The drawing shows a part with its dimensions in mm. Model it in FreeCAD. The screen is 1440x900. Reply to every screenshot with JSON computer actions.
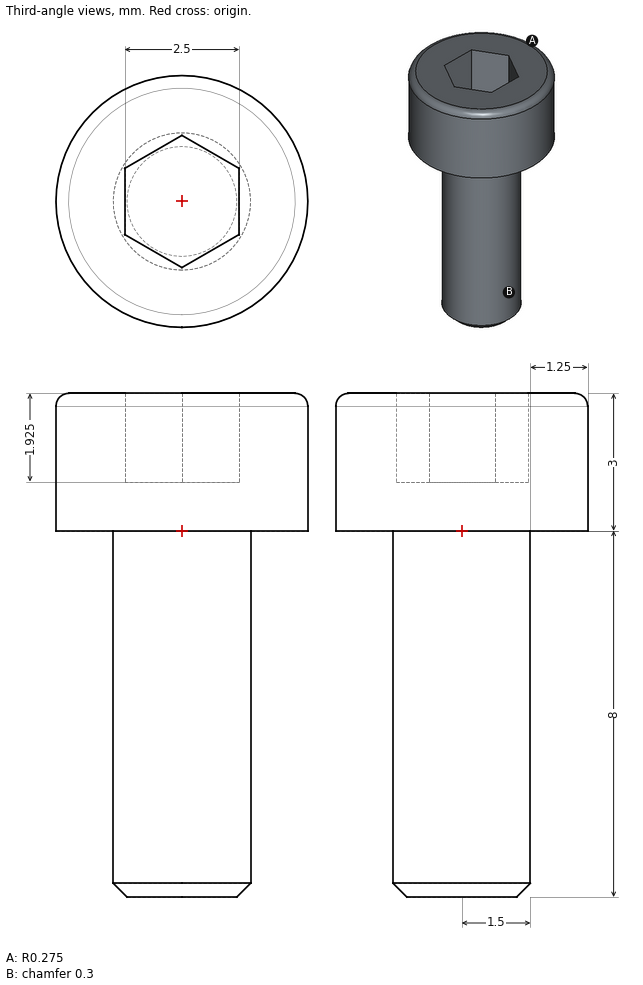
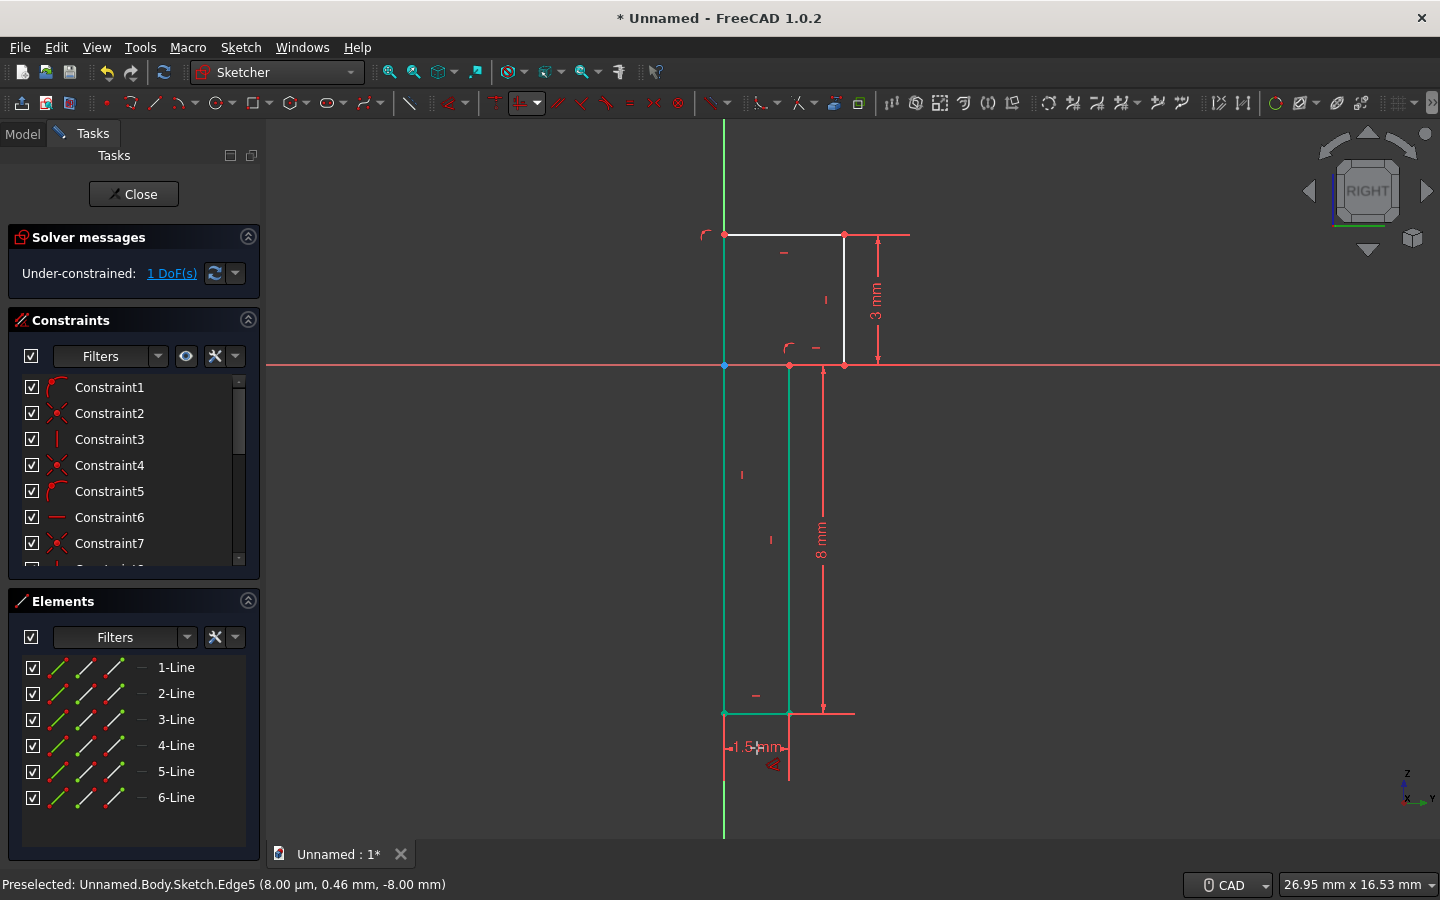
{"action": "left_click", "coordinate": [806, 365]}
{"action": "left_click", "coordinate": [817, 331]}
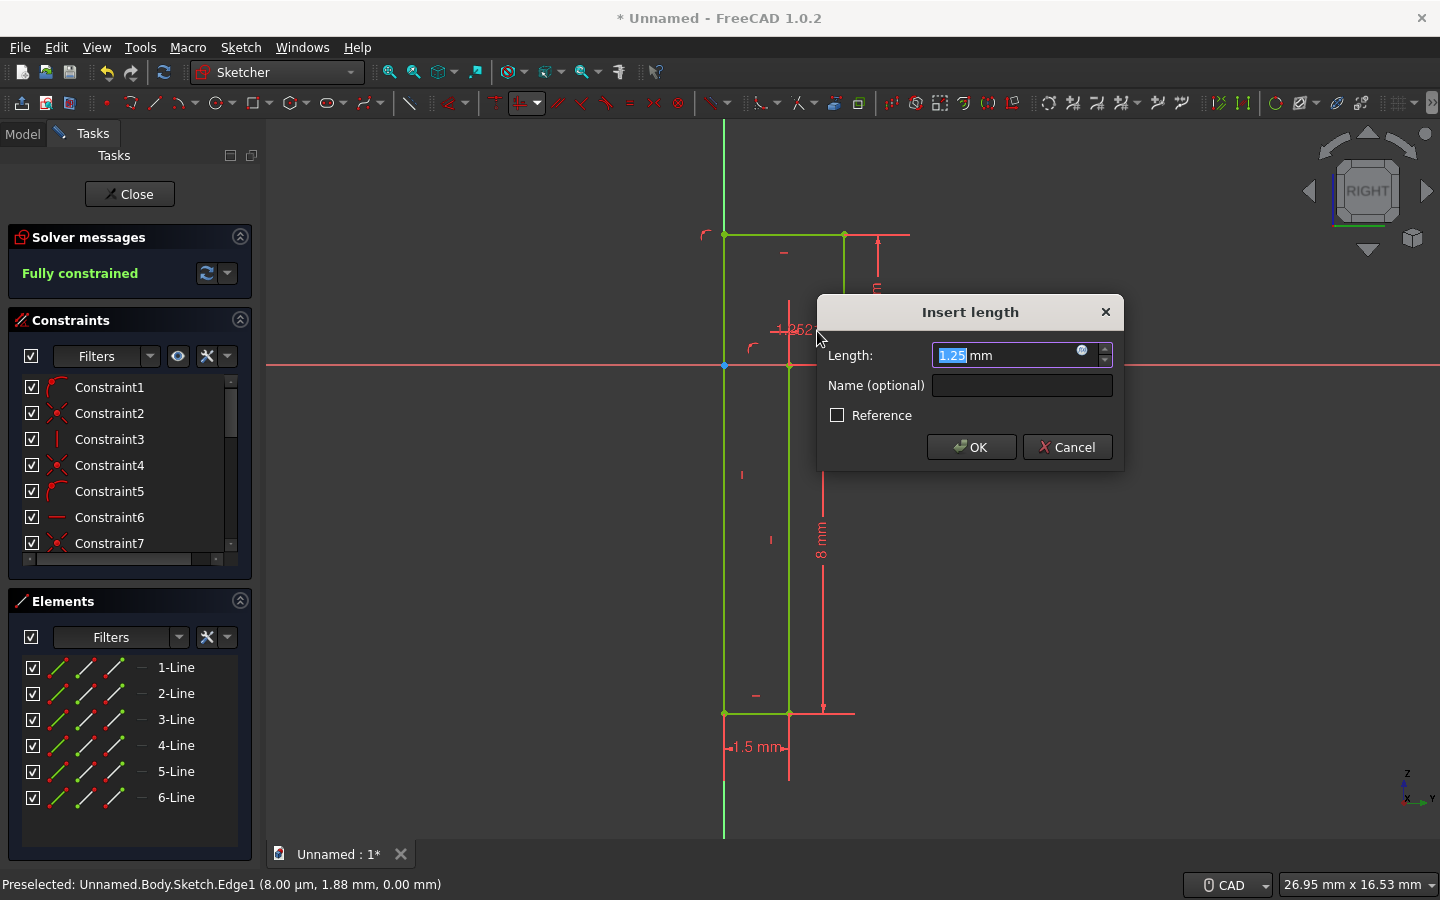
{"action": "type", "text": "1.25"}
{"action": "key", "text": "Return"}
{"action": "key", "text": "Escape"}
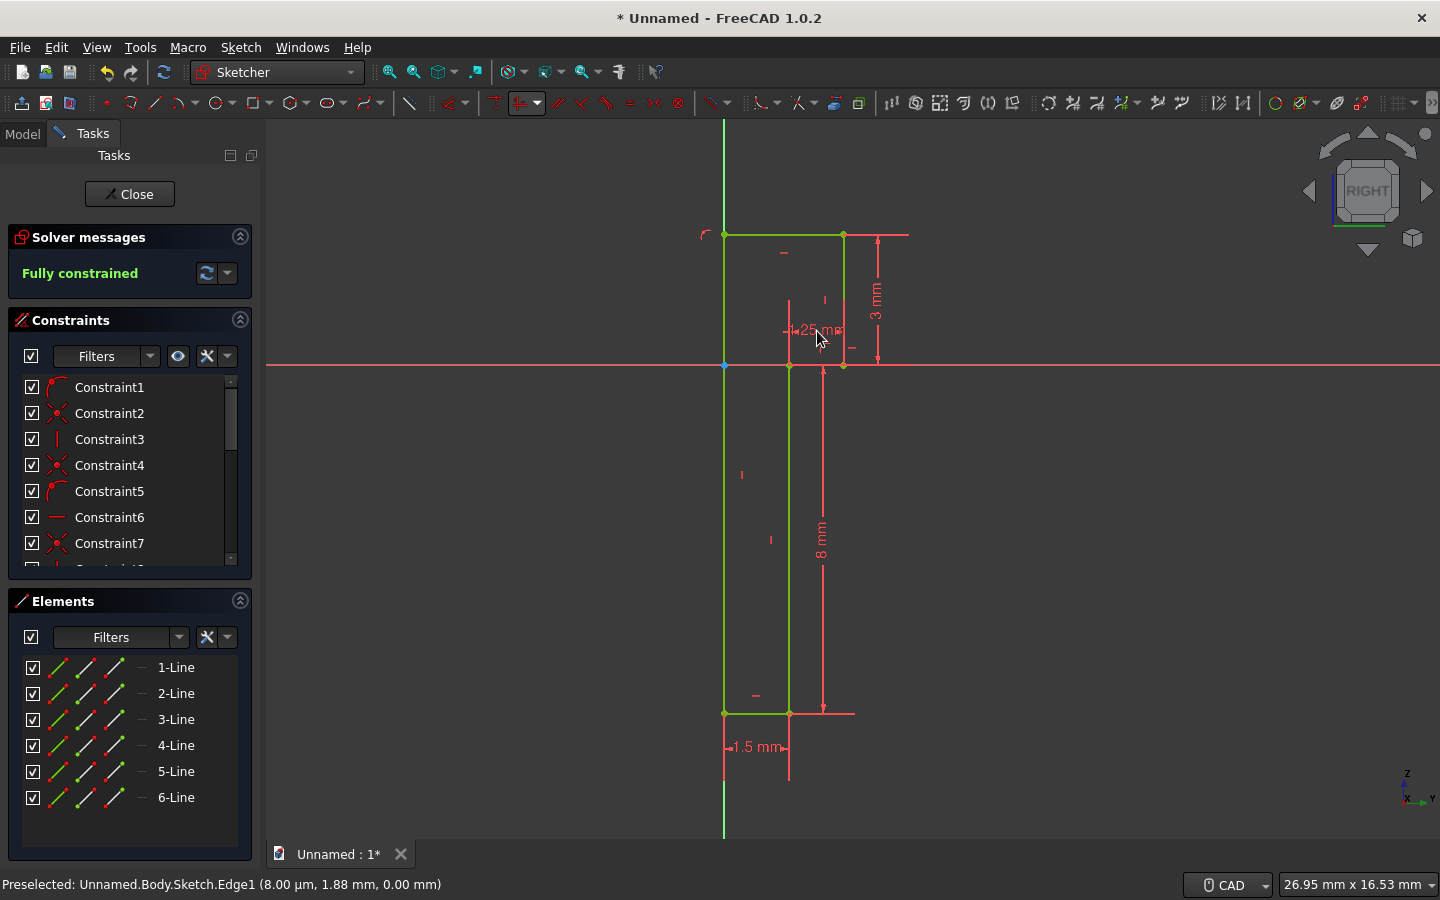
{"action": "left_click", "coordinate": [130, 194]}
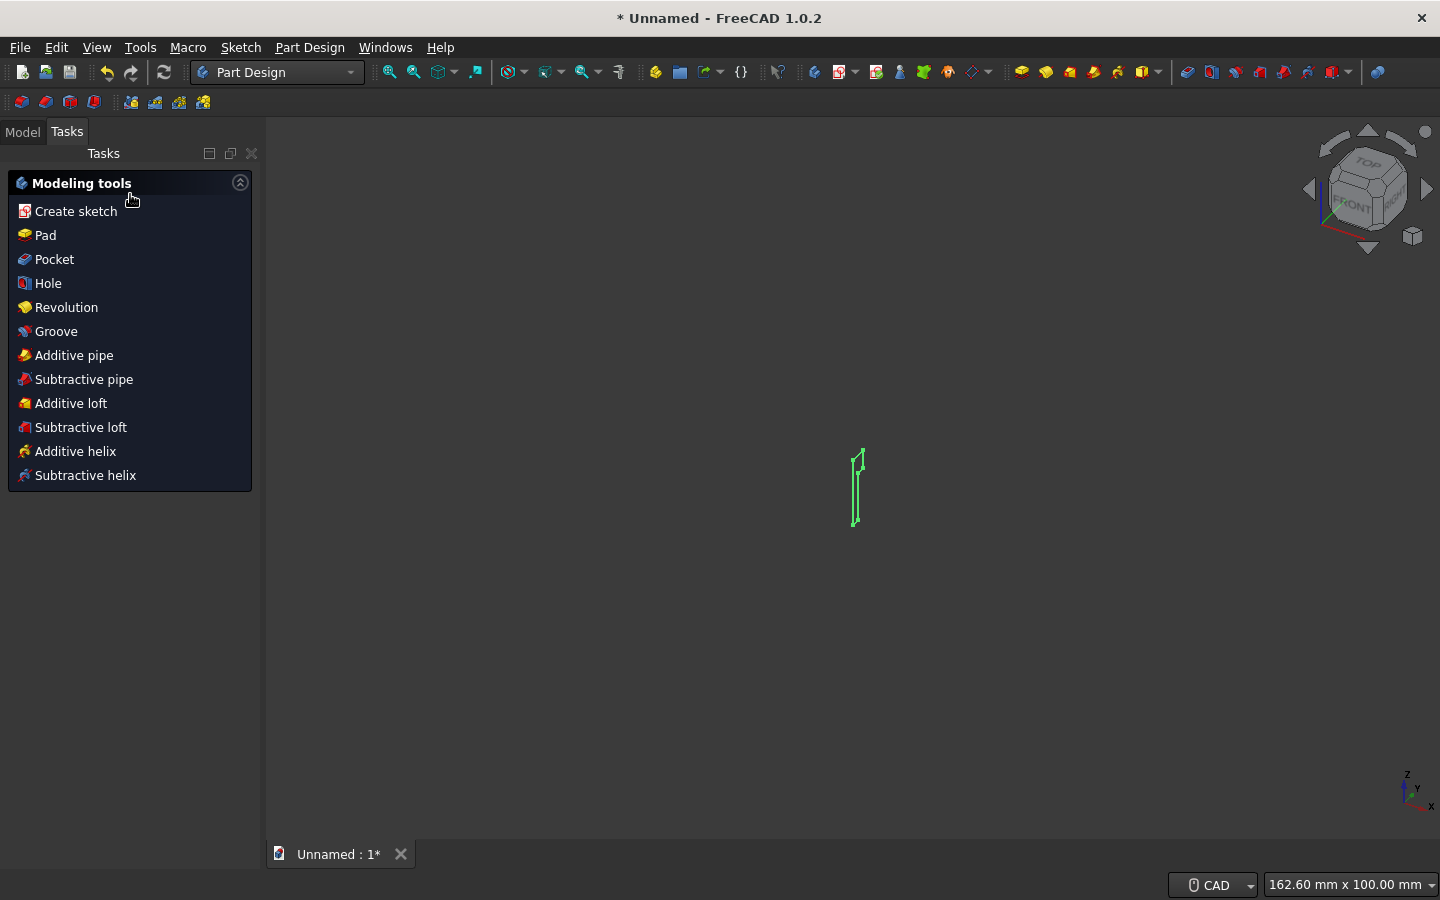
{"action": "left_click", "coordinate": [1046, 72]}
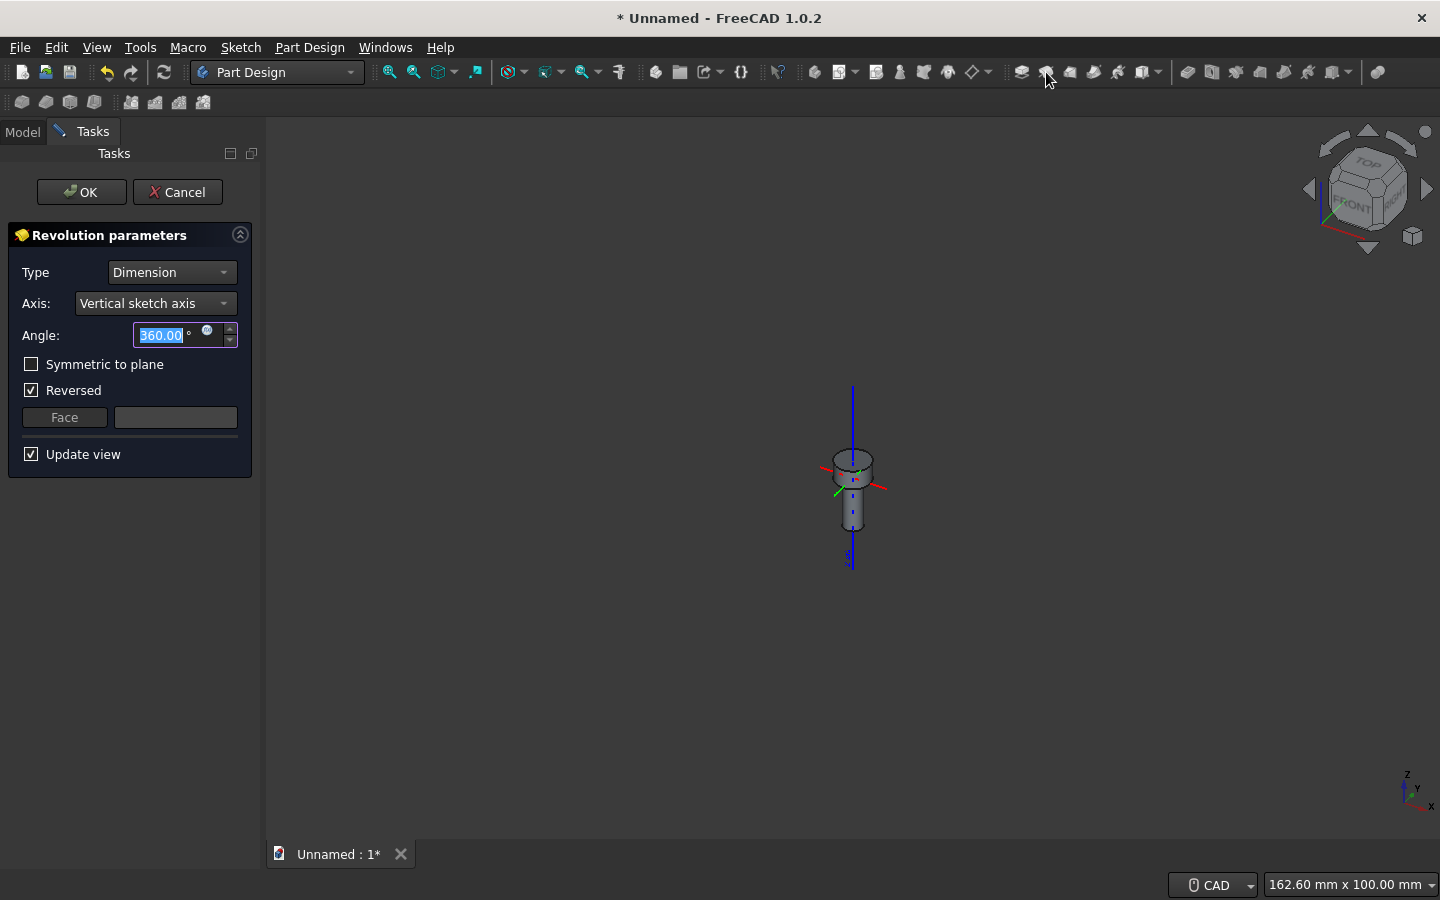
{"action": "left_click", "coordinate": [82, 192]}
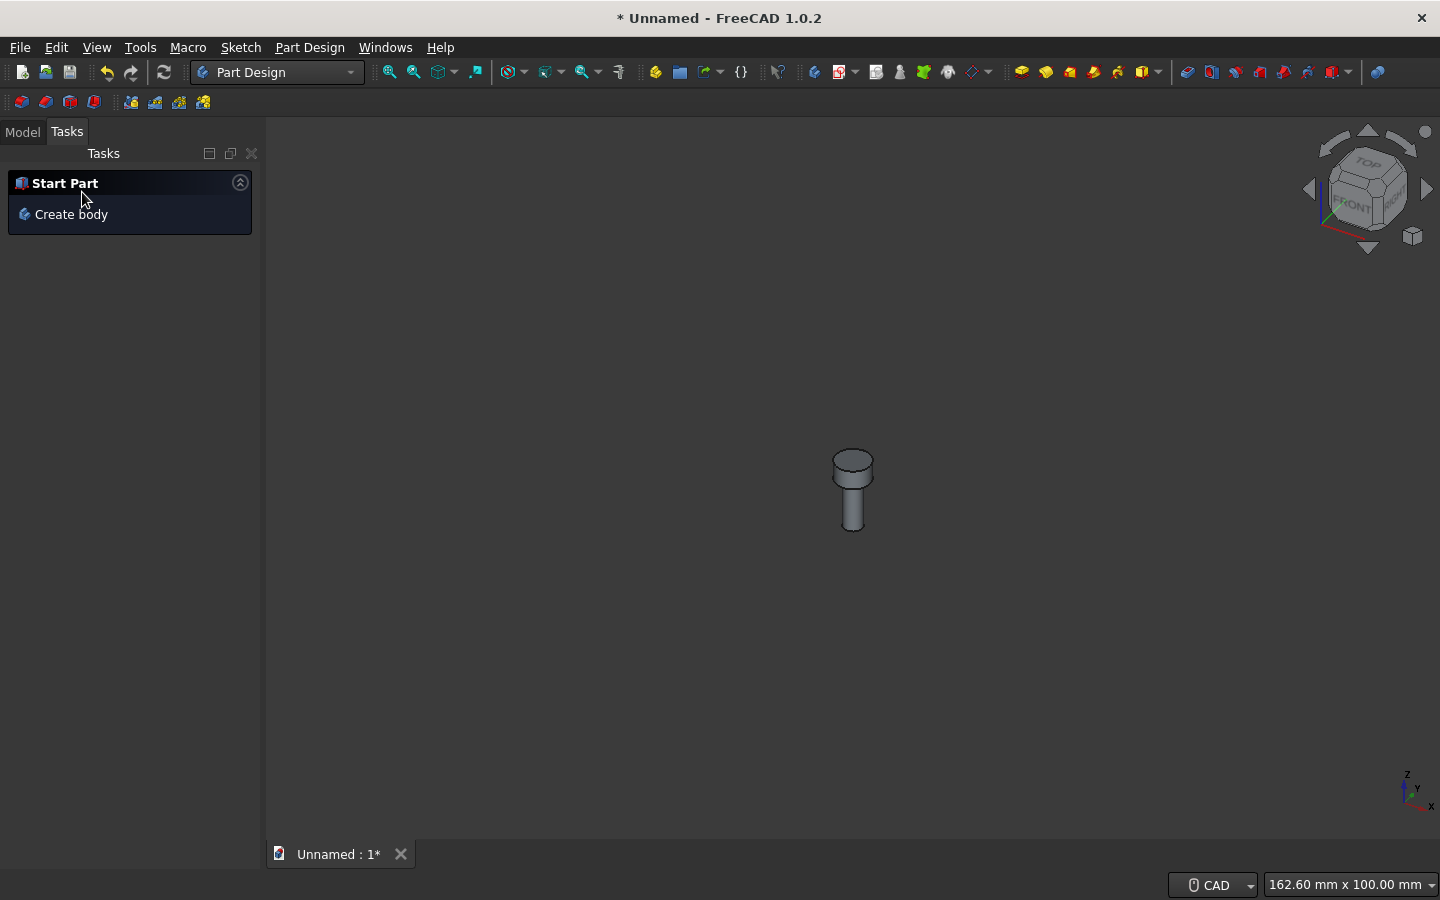
{"action": "left_click", "coordinate": [390, 72]}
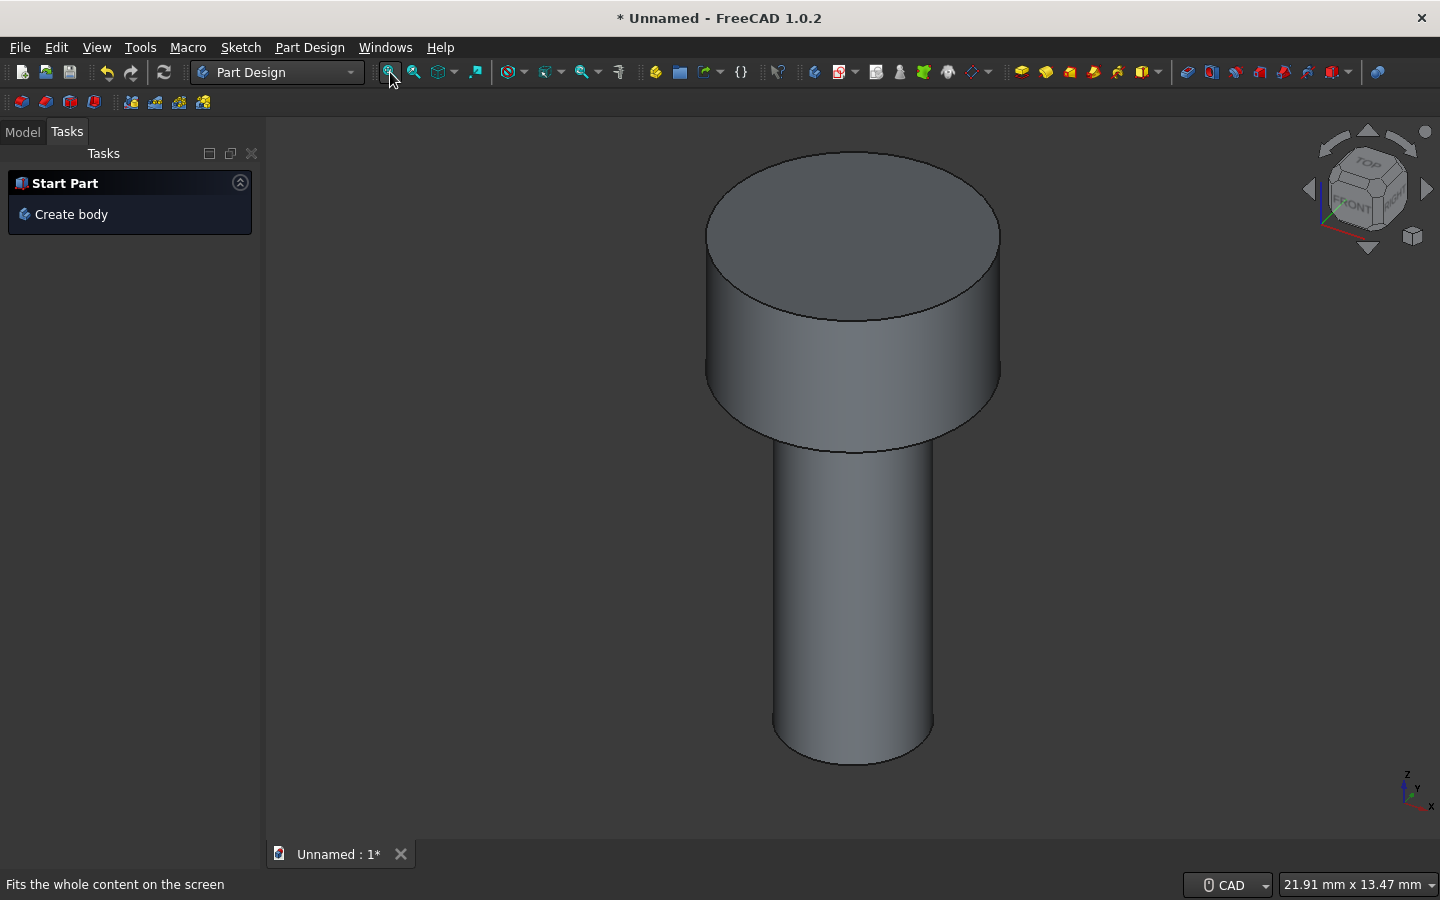
{"action": "left_click", "coordinate": [853, 236]}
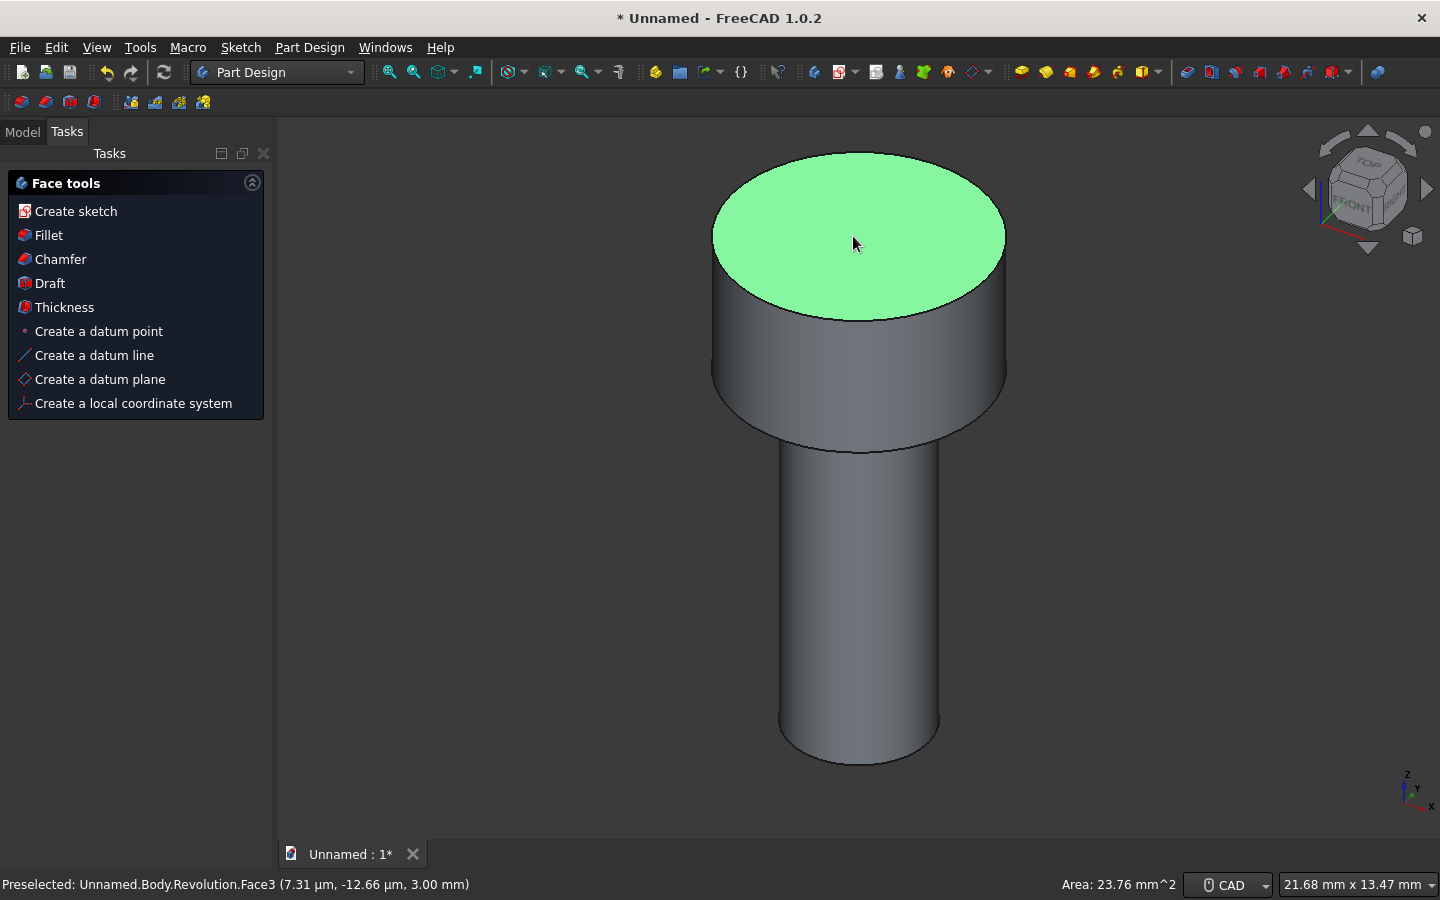
{"action": "left_click", "coordinate": [840, 72]}